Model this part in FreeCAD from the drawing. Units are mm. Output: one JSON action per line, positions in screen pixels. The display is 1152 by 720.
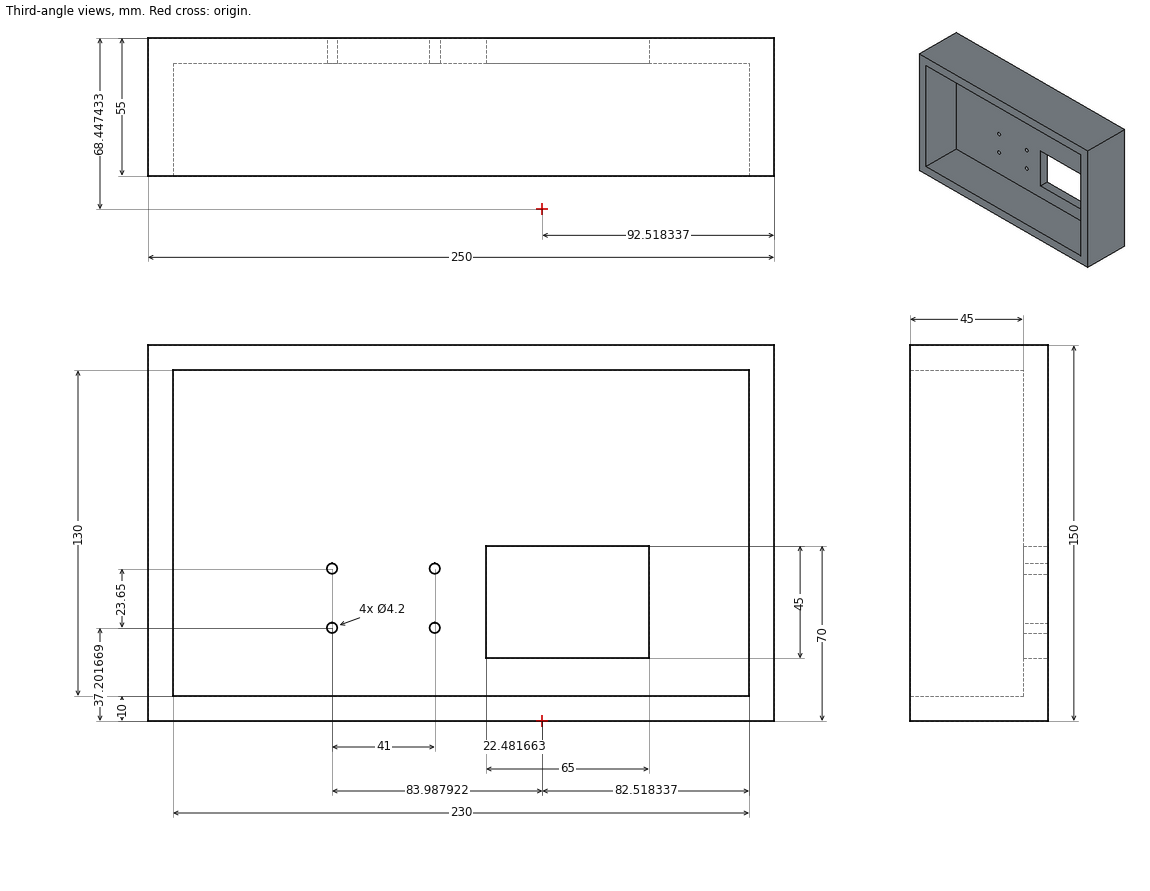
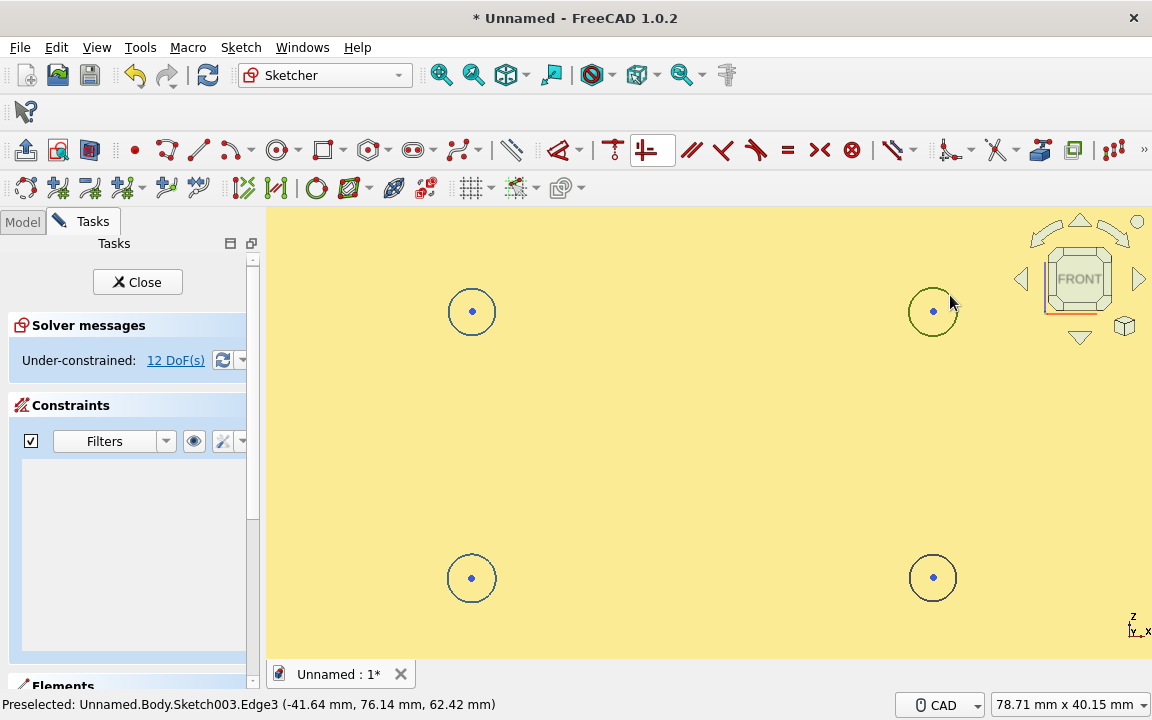
{"action": "left_click", "coordinate": [949, 561]}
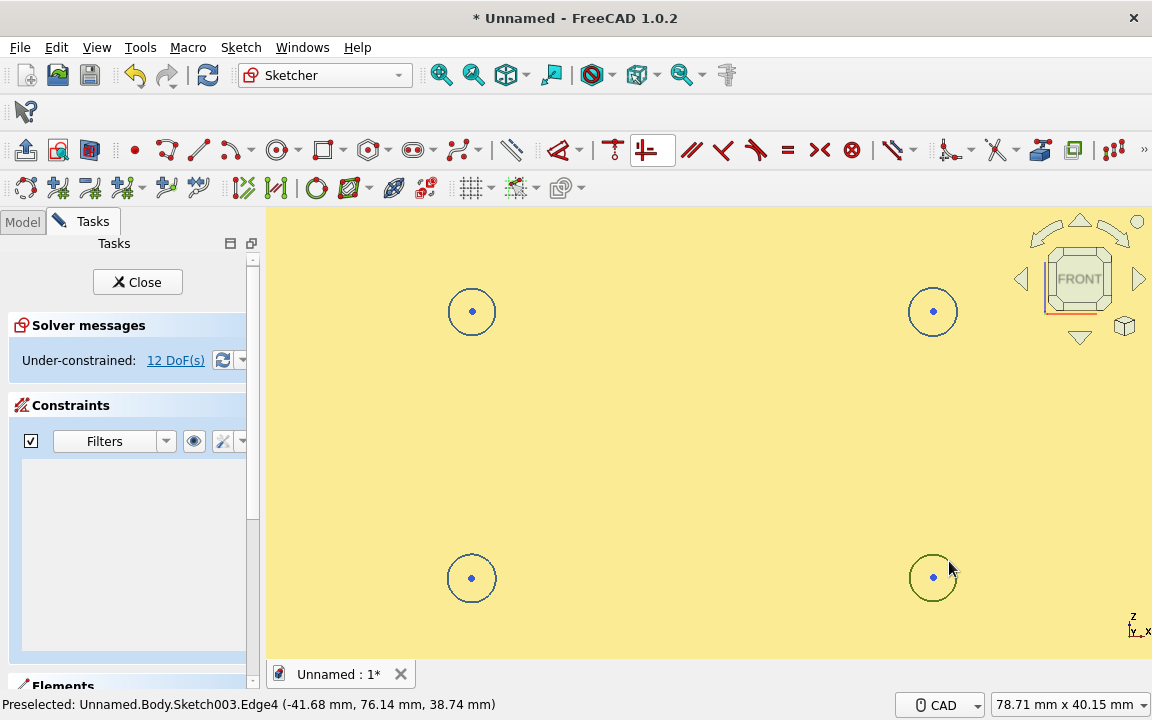
{"action": "left_click", "coordinate": [788, 150]}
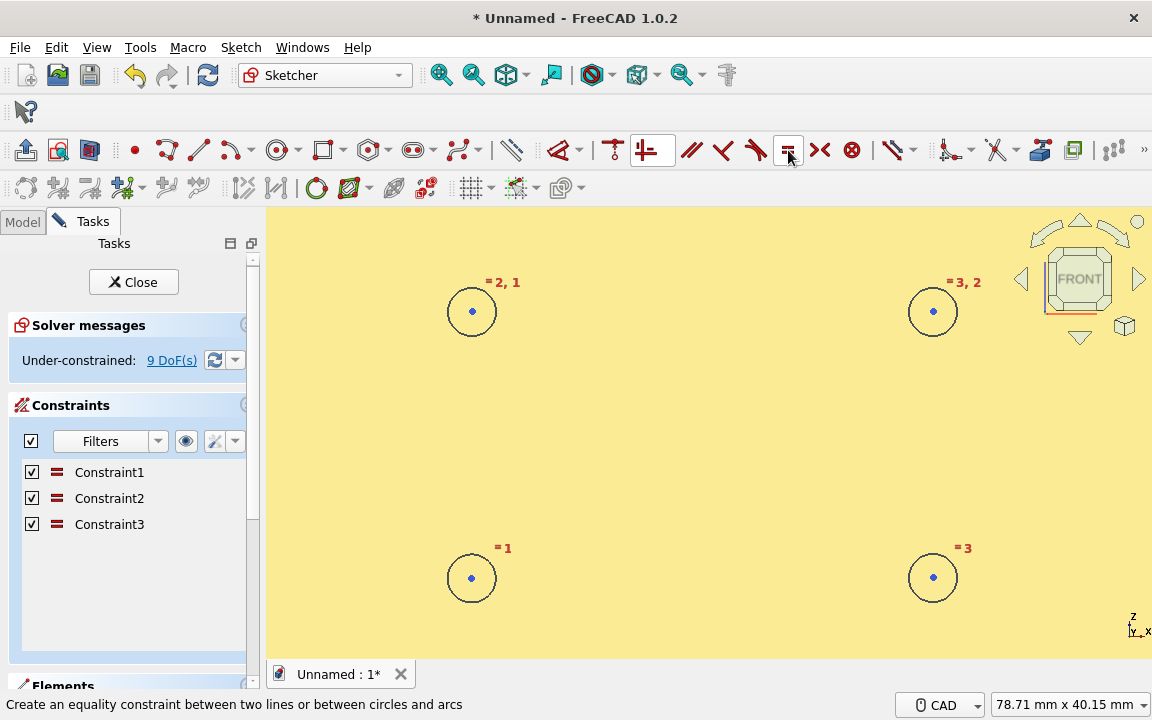
{"action": "left_click", "coordinate": [472, 578]}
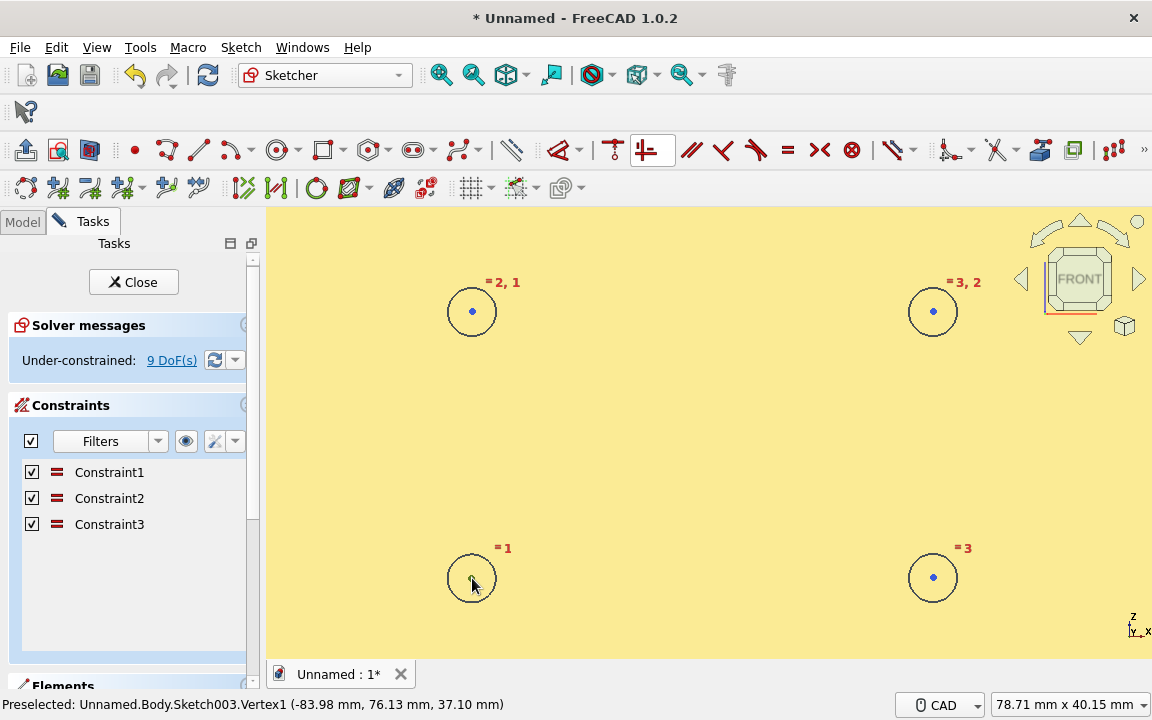
{"action": "left_click", "coordinate": [472, 312]}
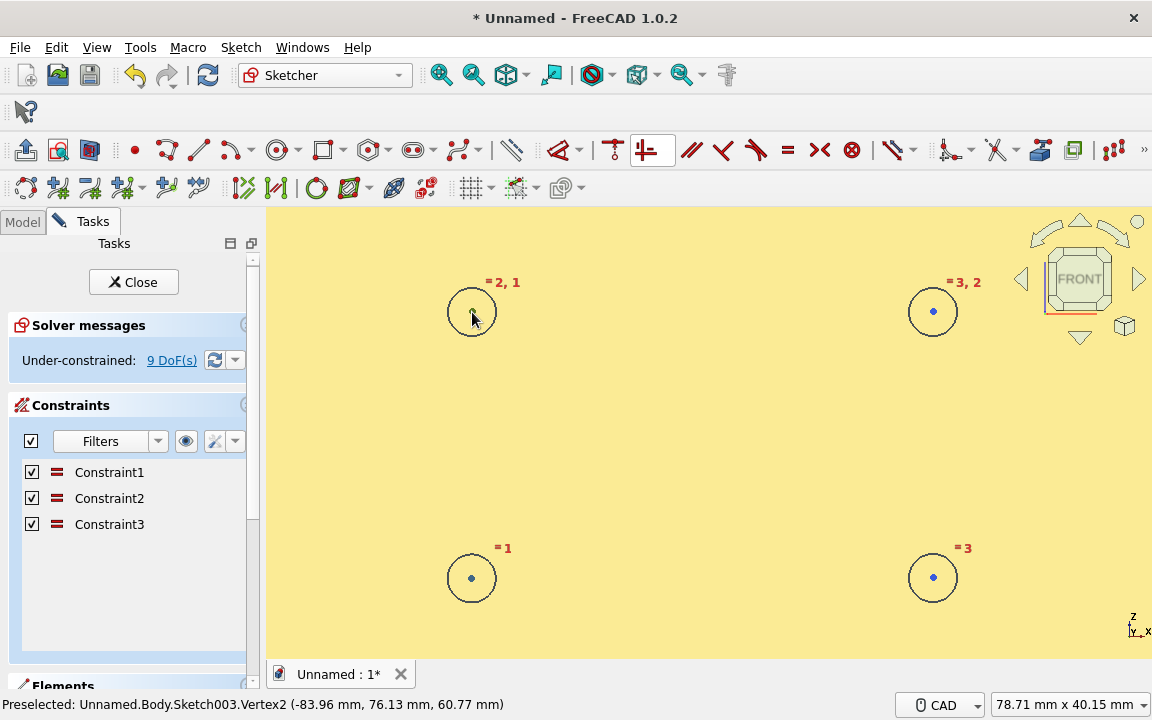
{"action": "key", "text": "v"}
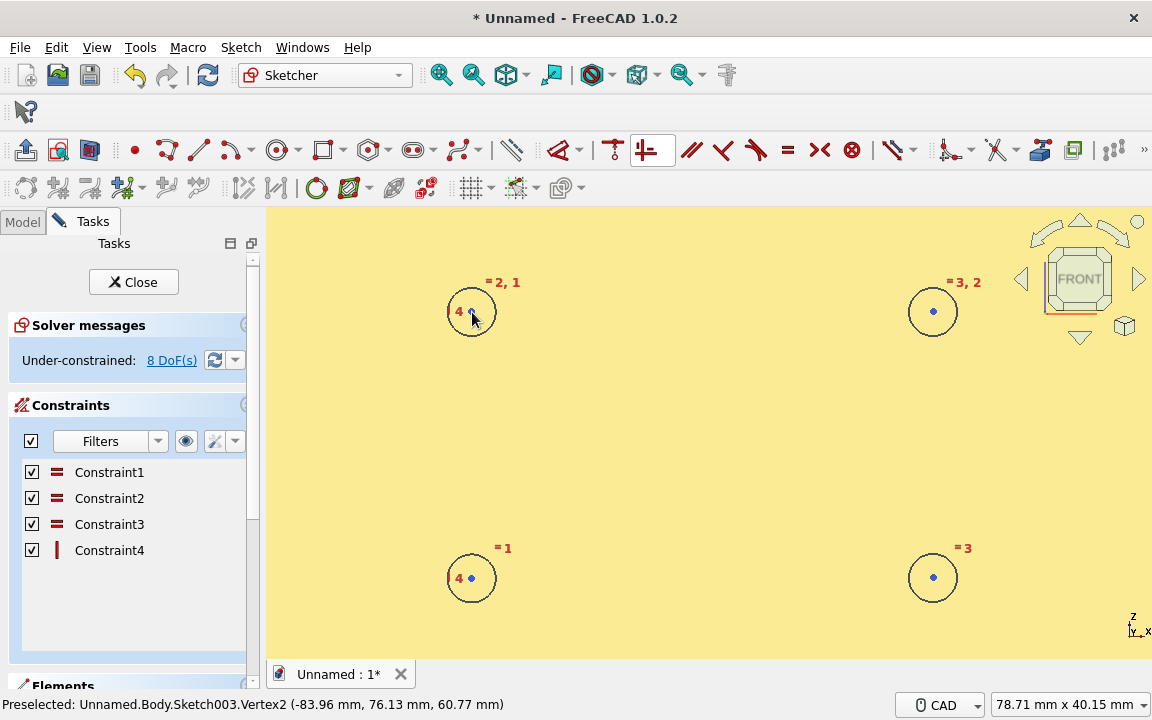
{"action": "left_click", "coordinate": [472, 312]}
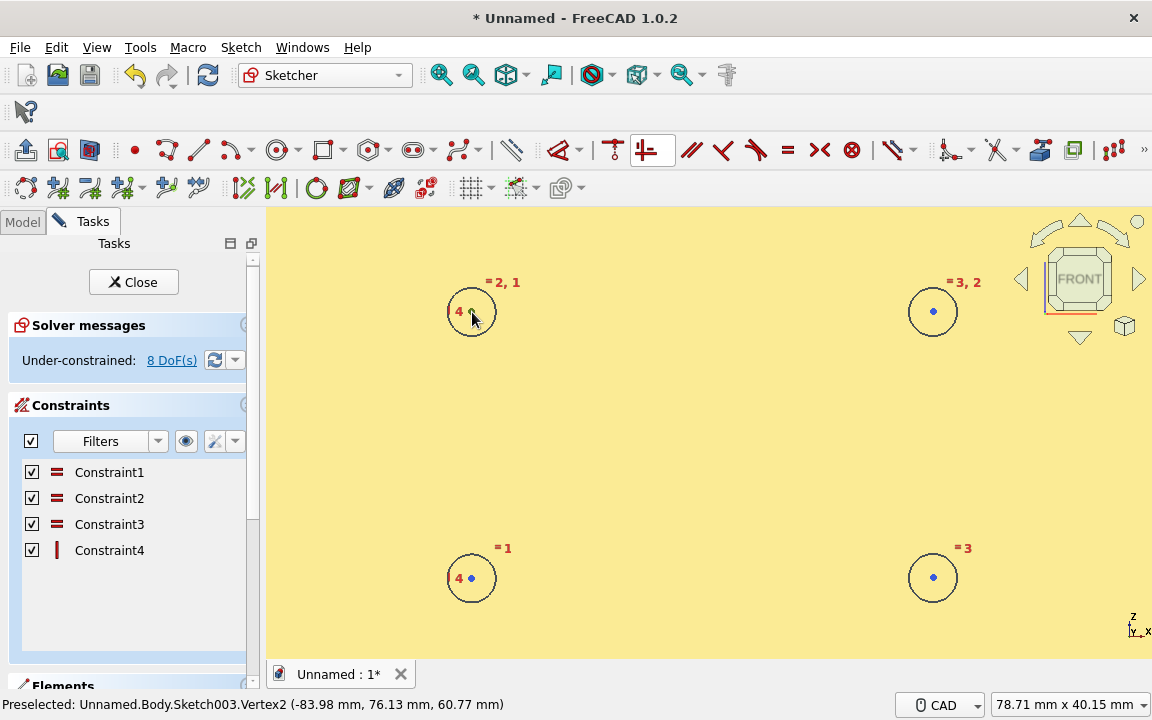
{"action": "left_click", "coordinate": [933, 312]}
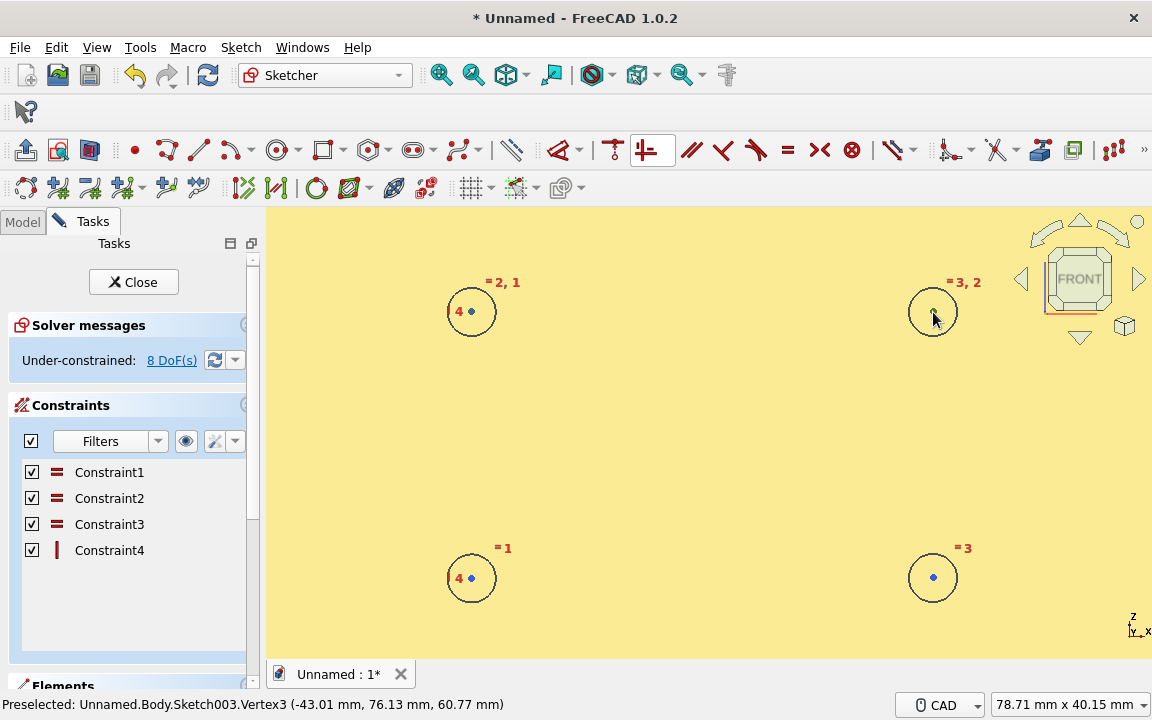
{"action": "left_click", "coordinate": [670, 150]}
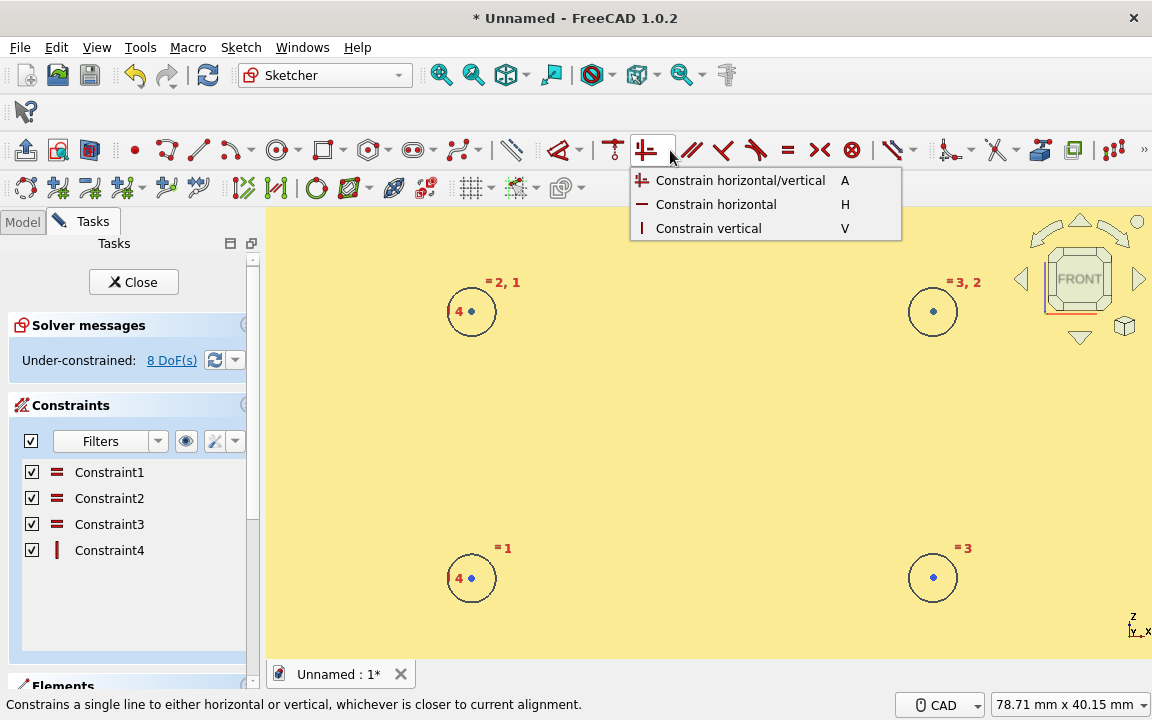
{"action": "left_click", "coordinate": [766, 204]}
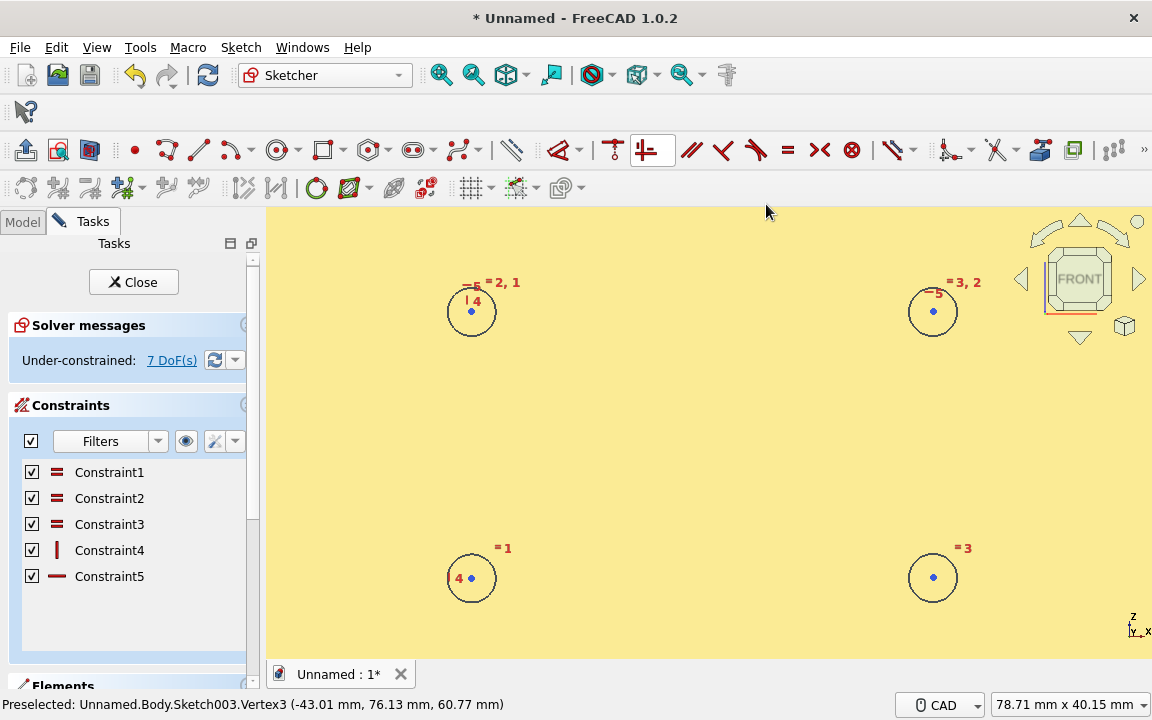
{"action": "left_click", "coordinate": [933, 312]}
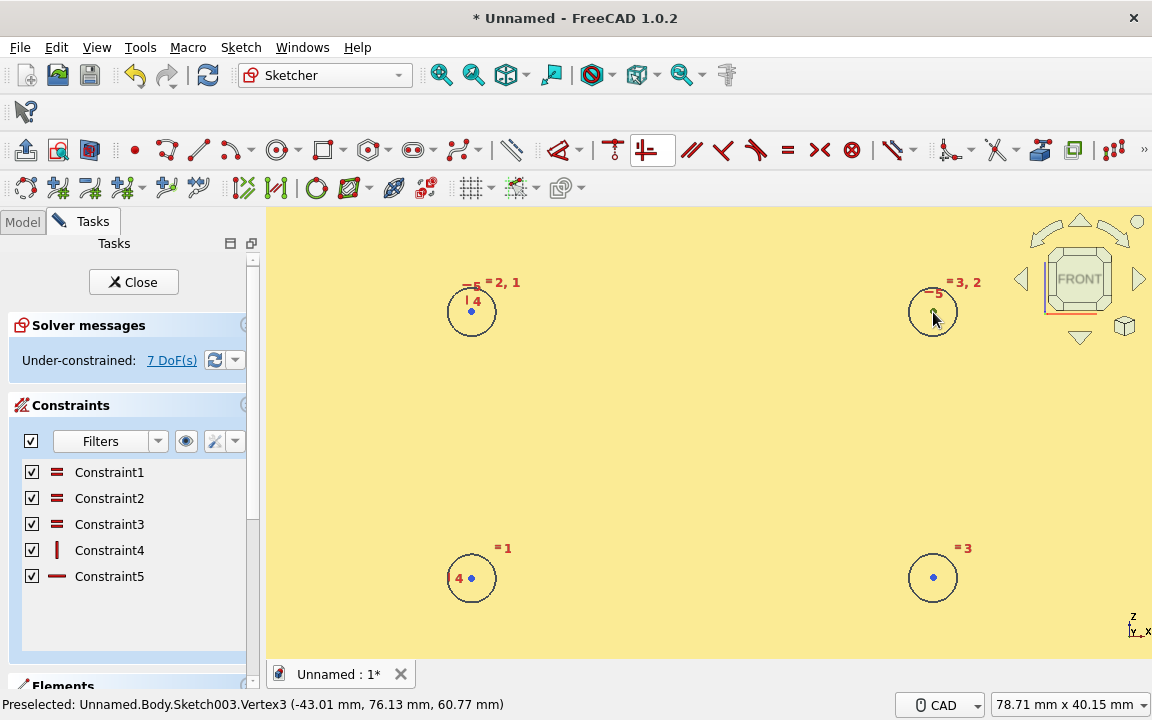
{"action": "left_click", "coordinate": [933, 578]}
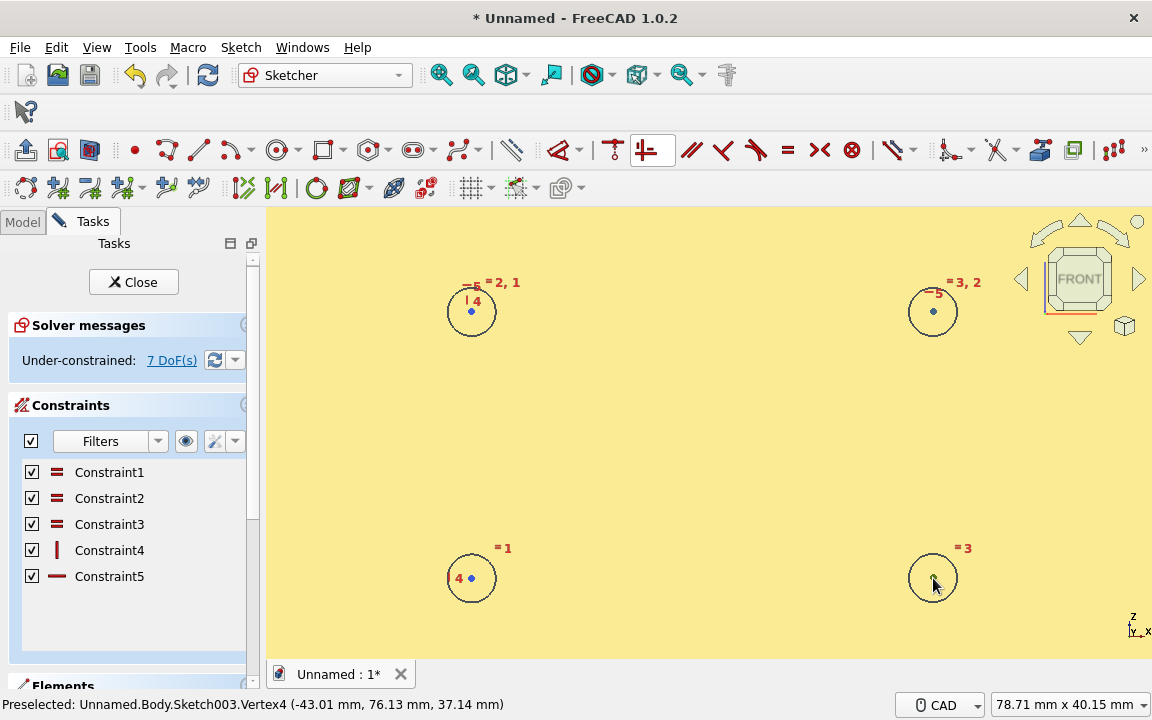
{"action": "left_click", "coordinate": [670, 150]}